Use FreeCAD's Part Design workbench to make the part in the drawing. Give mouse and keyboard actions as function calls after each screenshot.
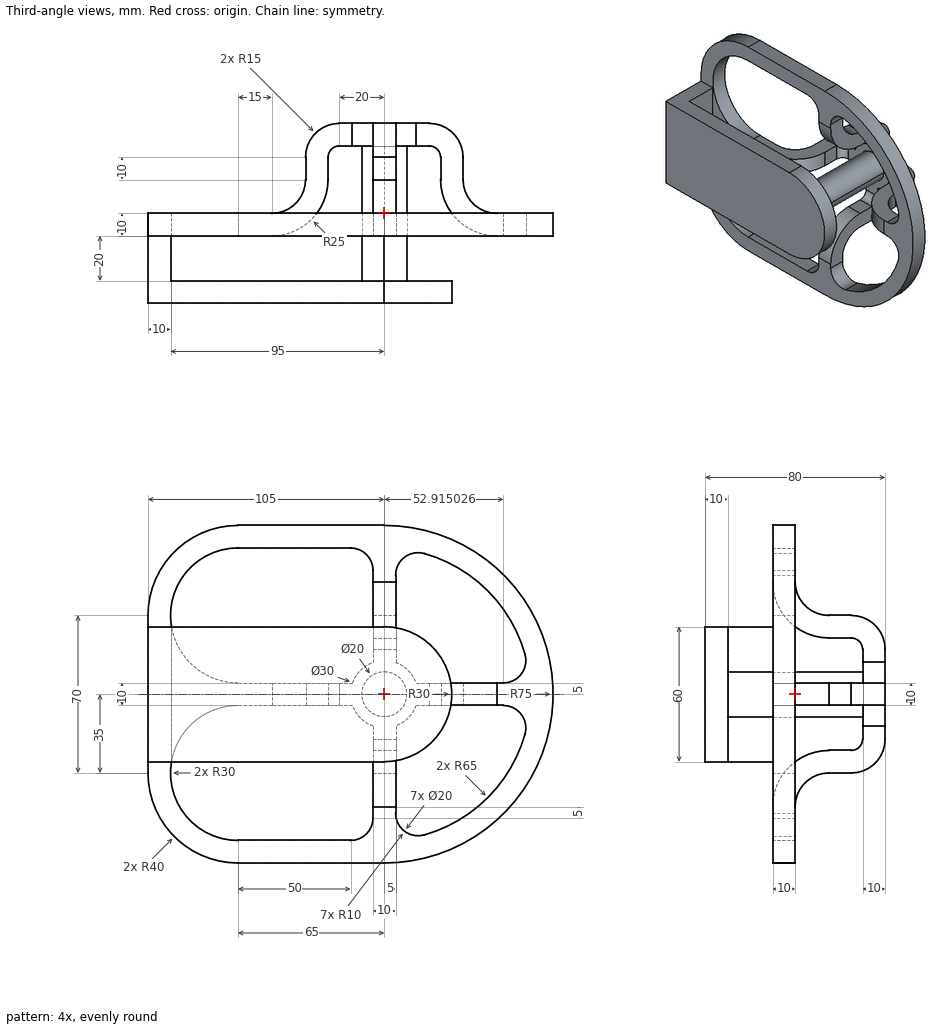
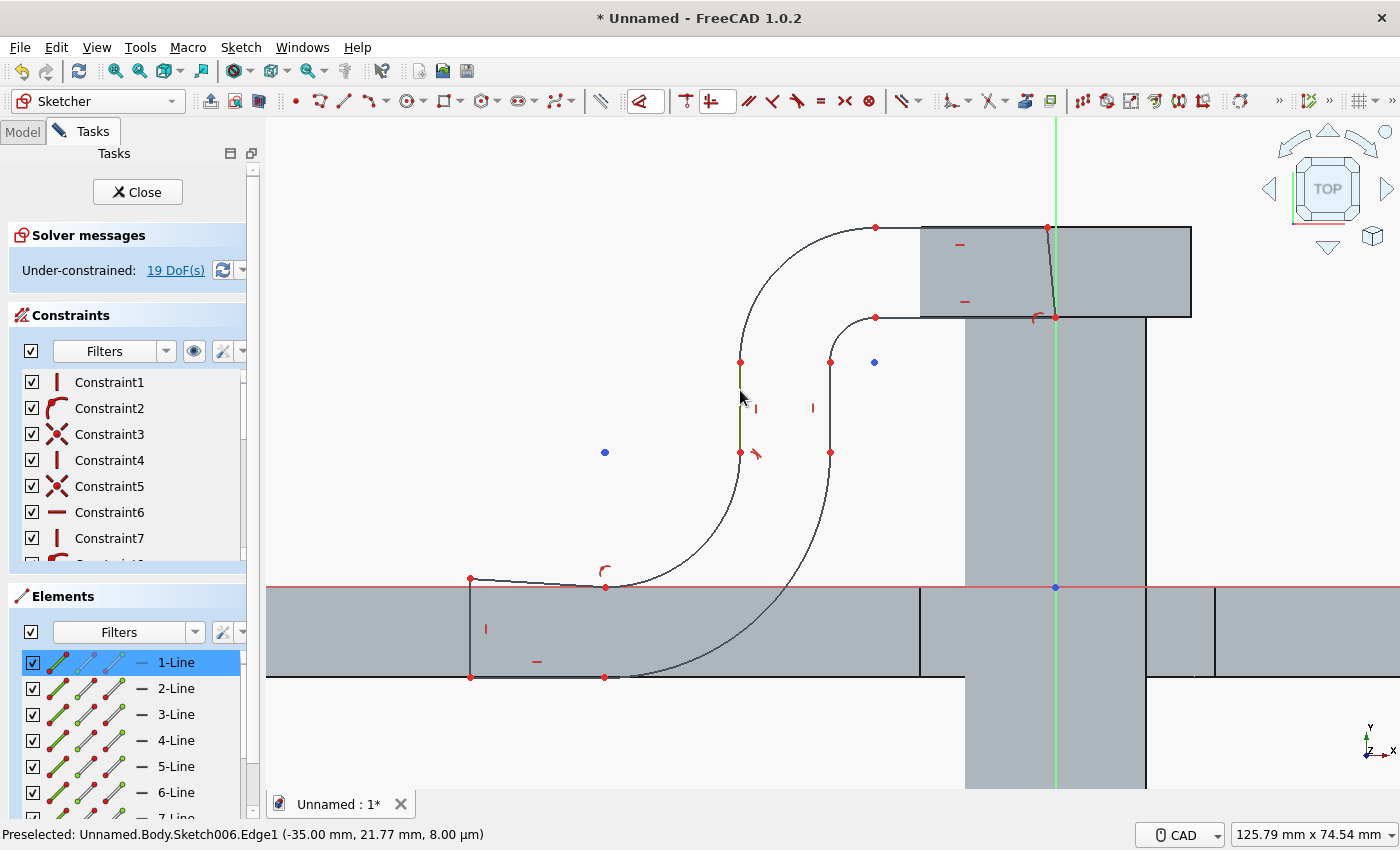
click(814, 243)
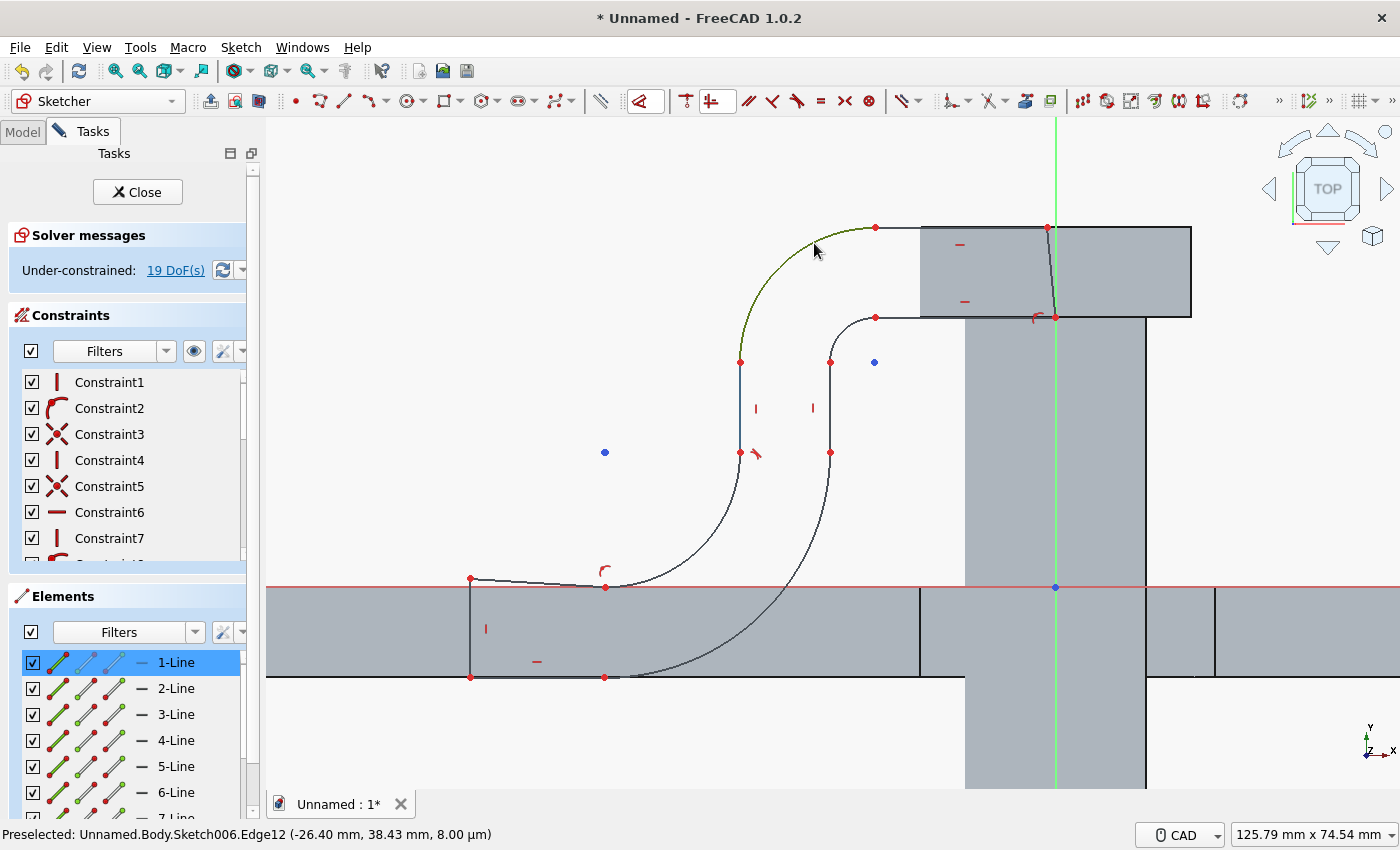
click(798, 102)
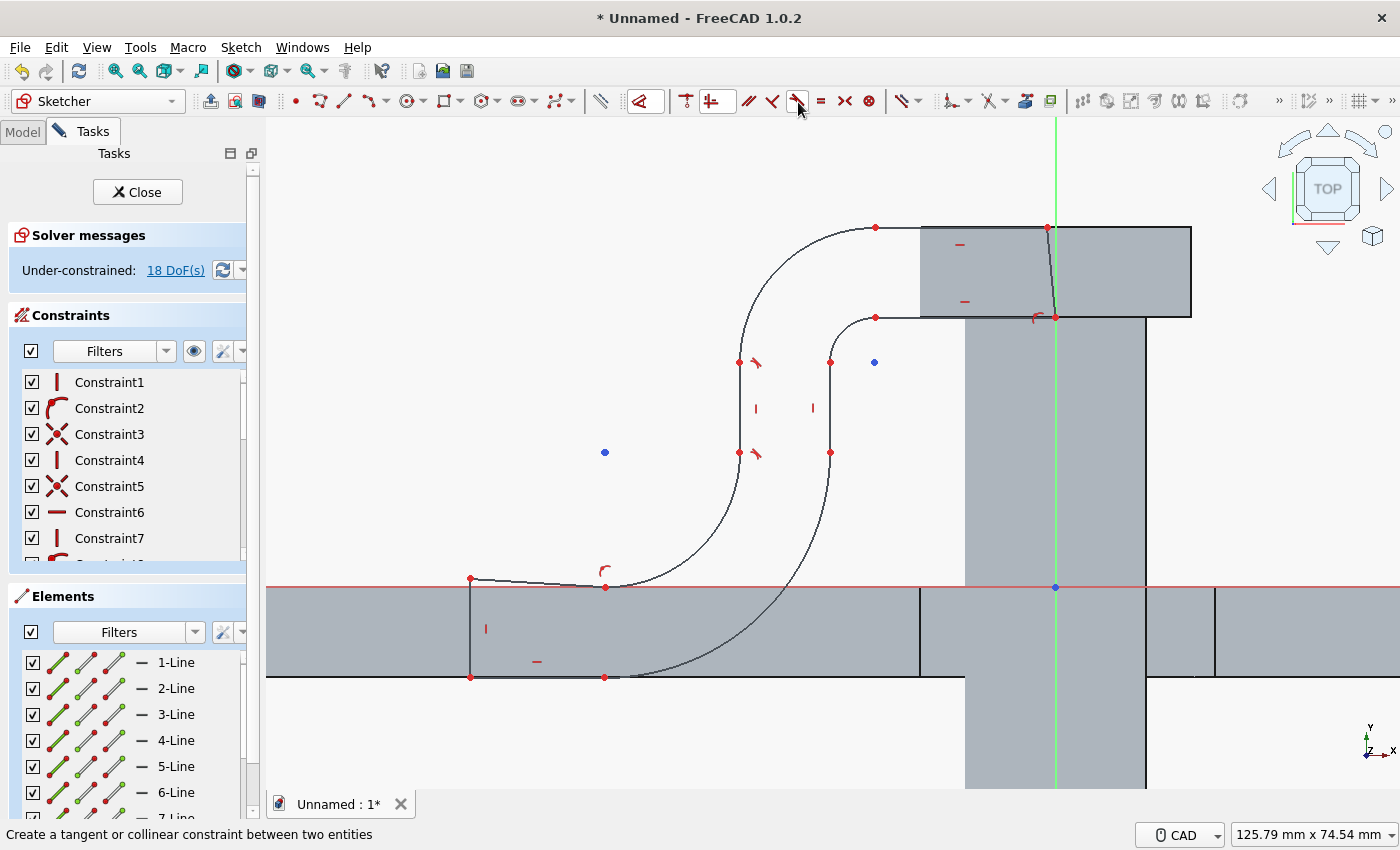
click(564, 585)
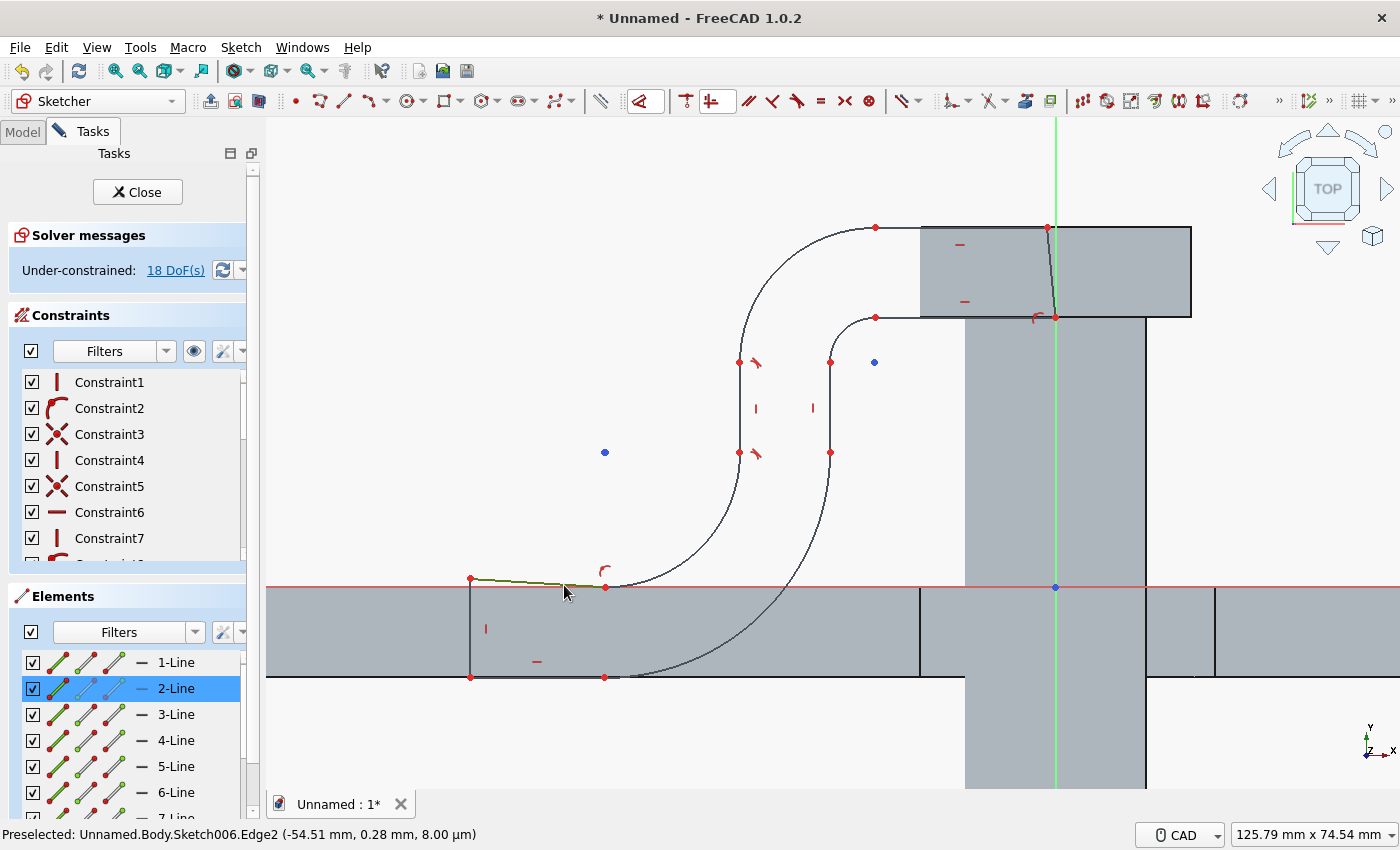
click(666, 573)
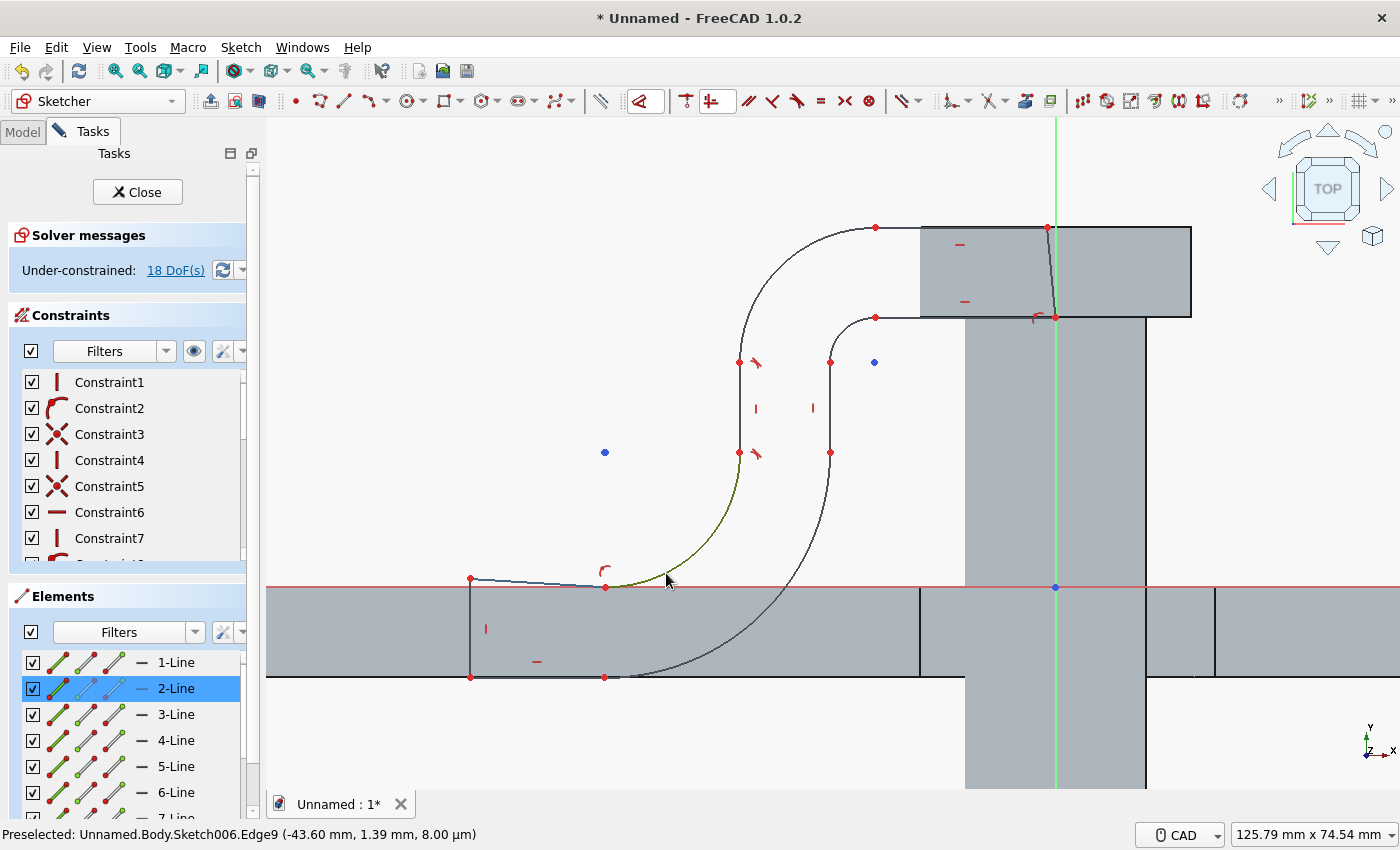
click(798, 102)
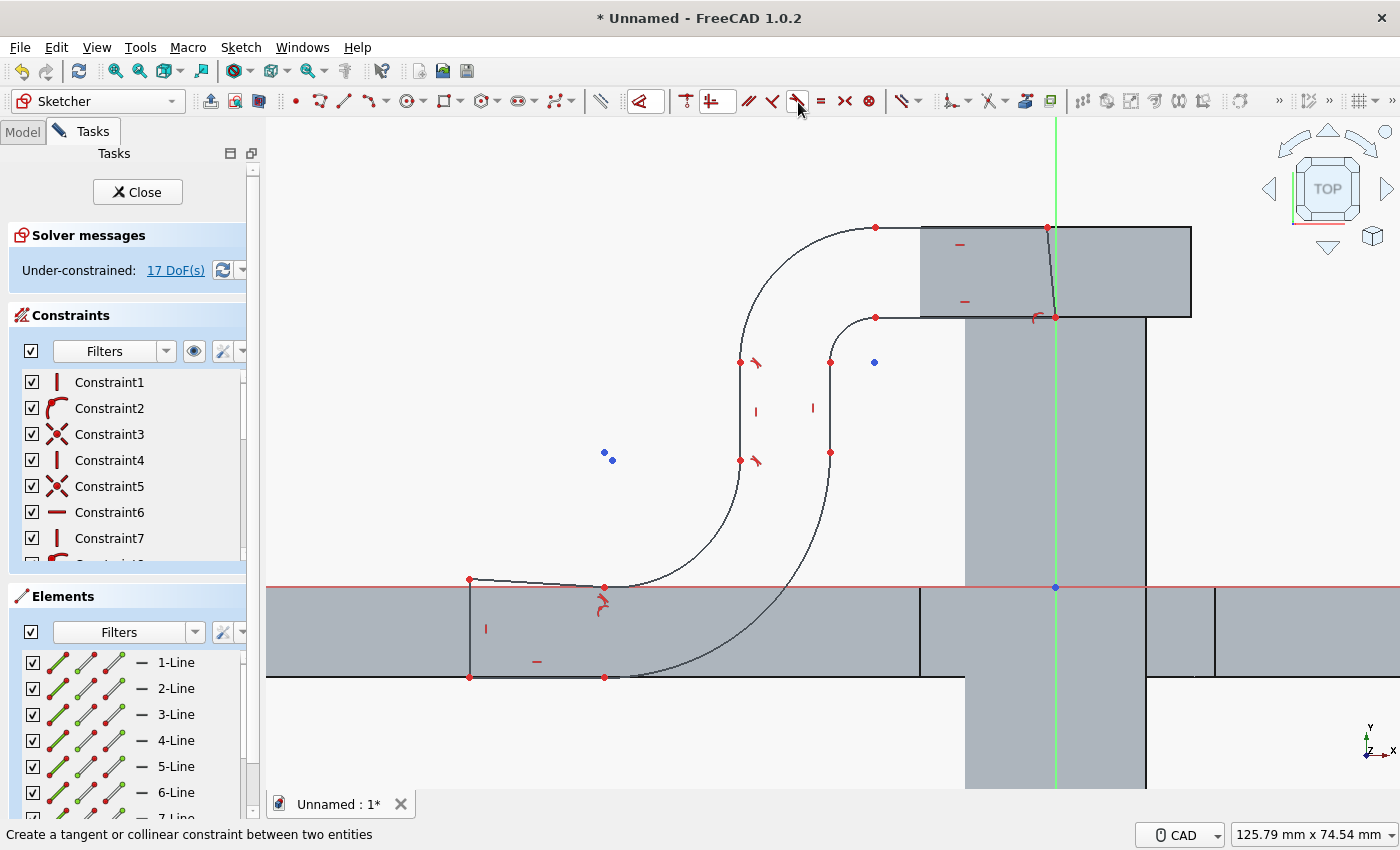
click(510, 678)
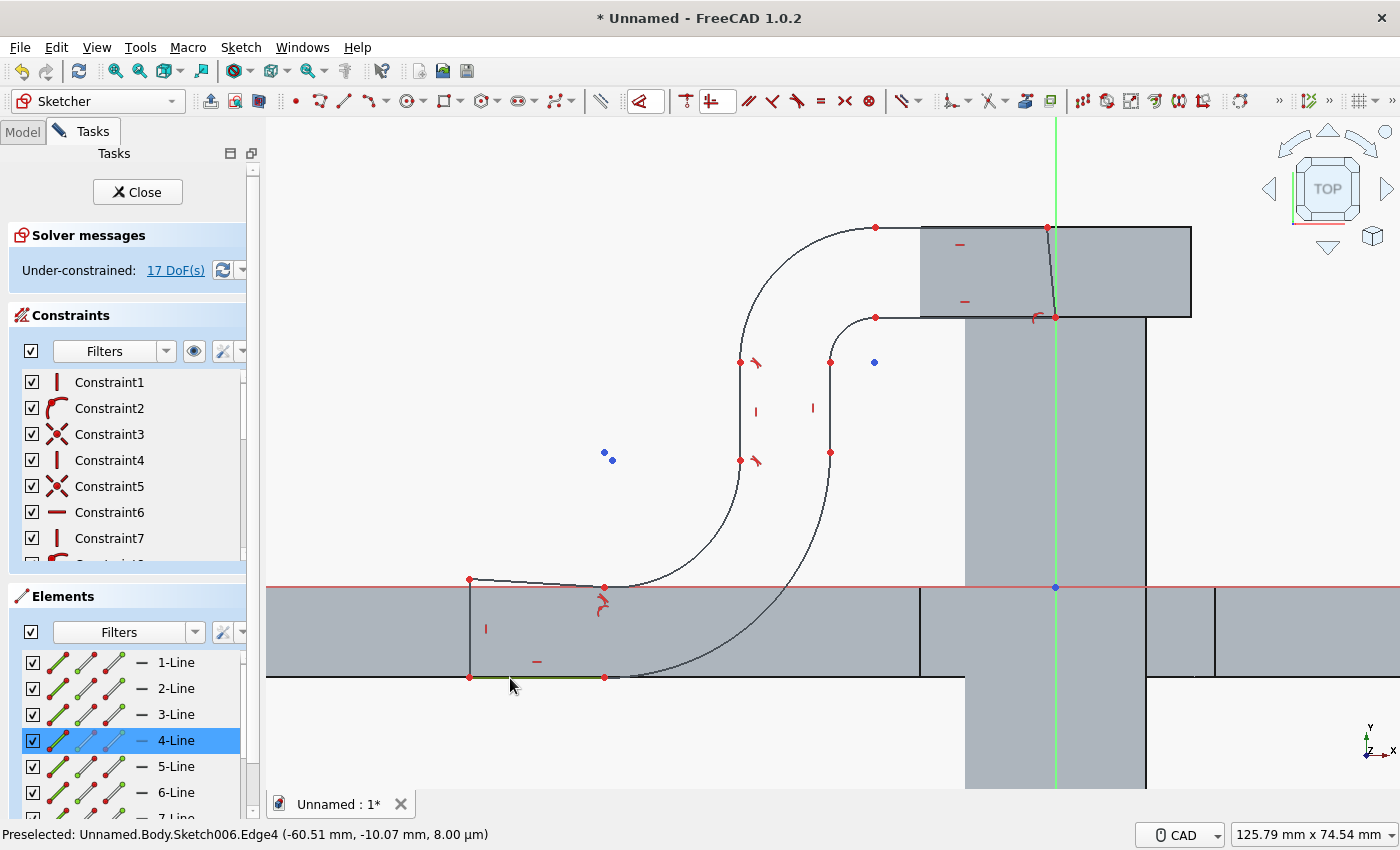
click(707, 653)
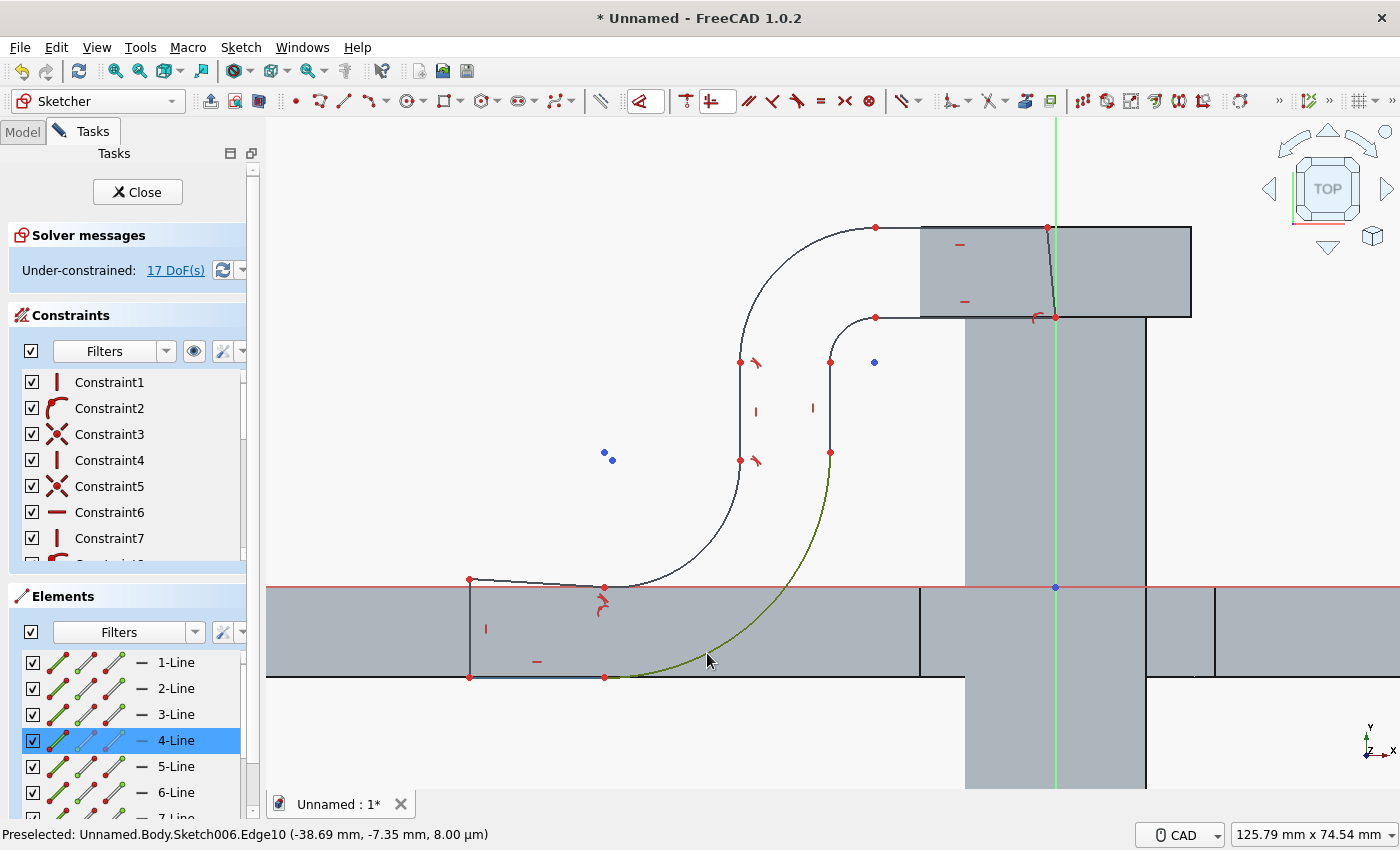
click(798, 102)